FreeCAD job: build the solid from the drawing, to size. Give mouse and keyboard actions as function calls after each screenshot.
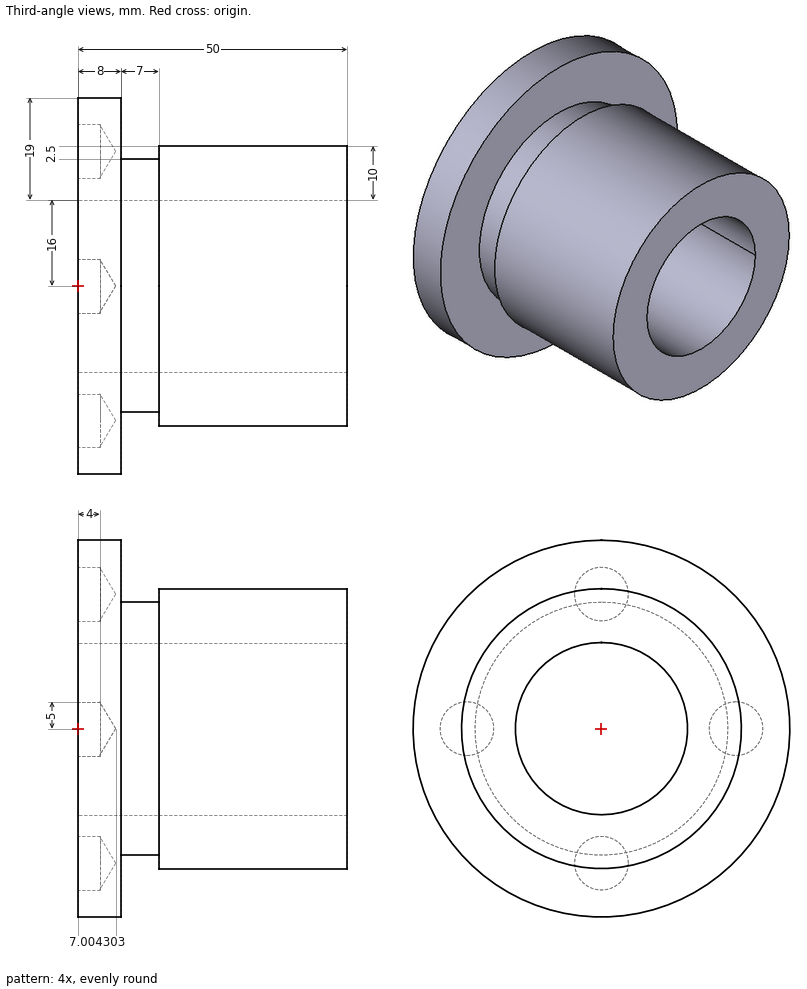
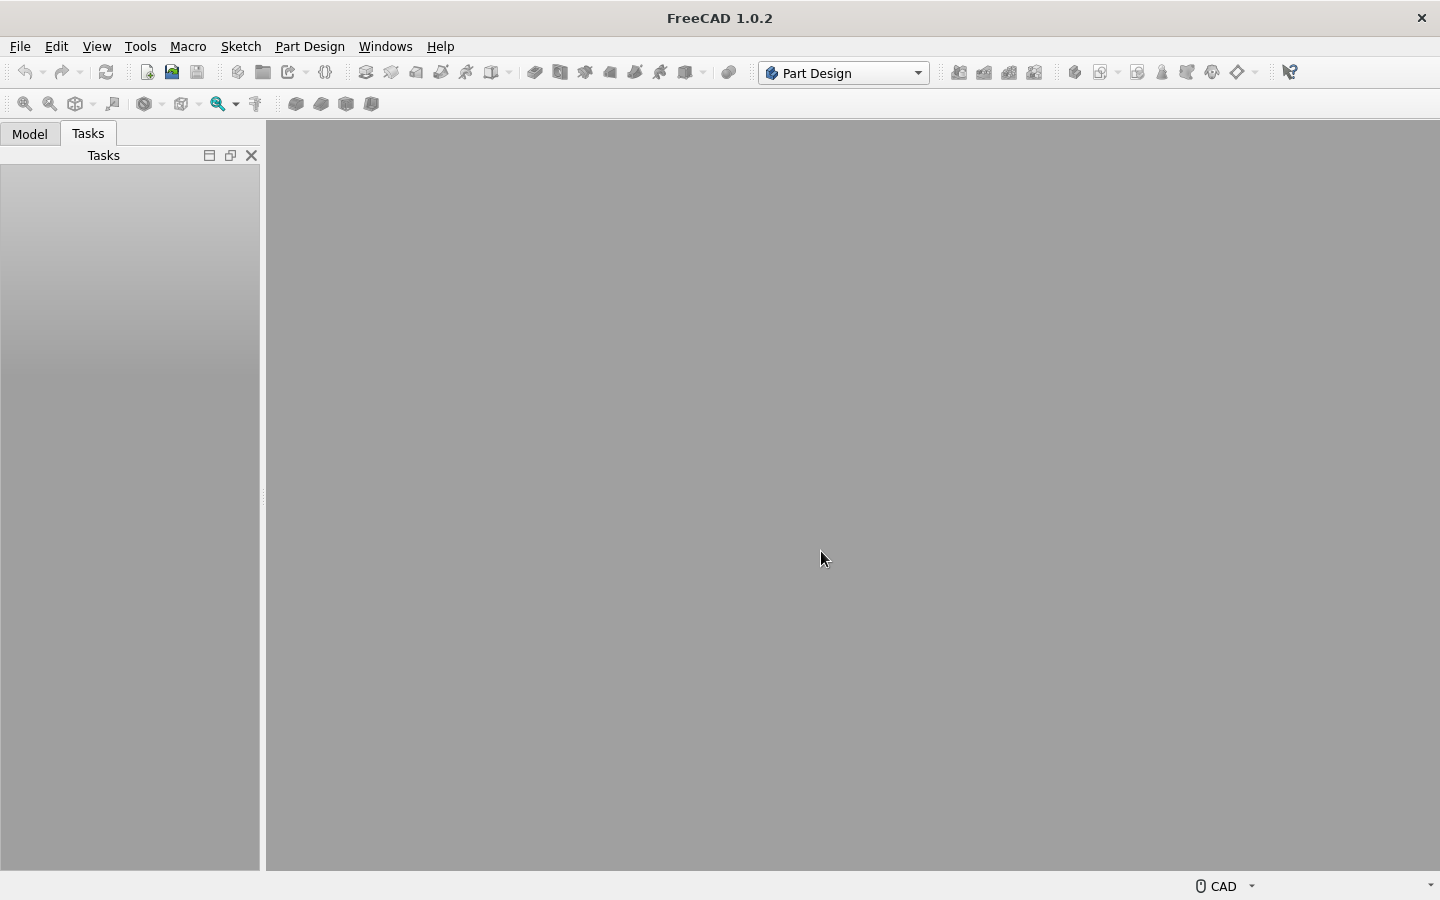
key(ctrl+n)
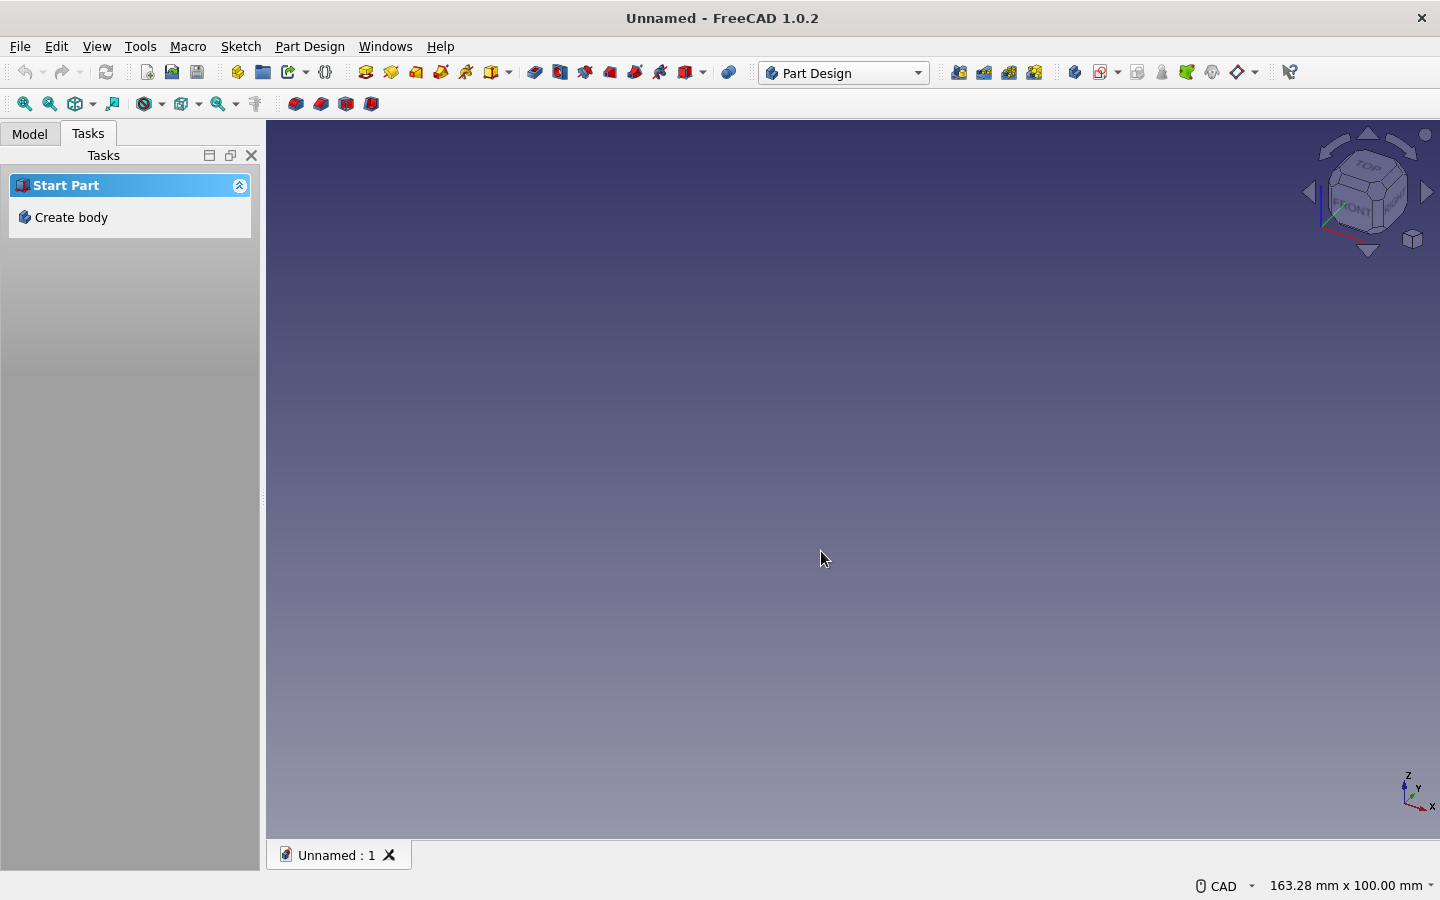
click(1100, 72)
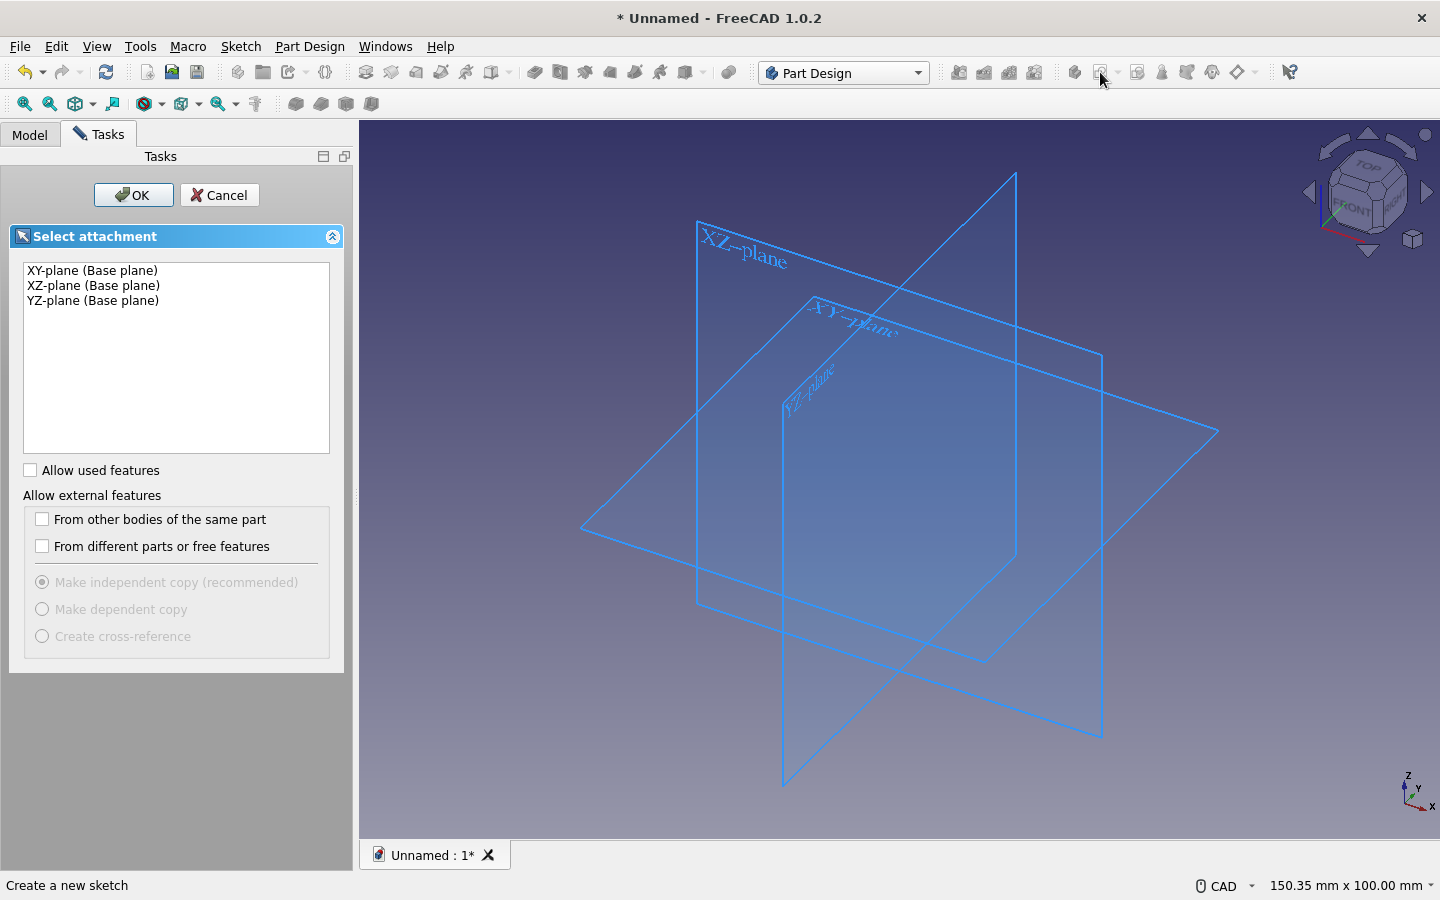
click(84, 270)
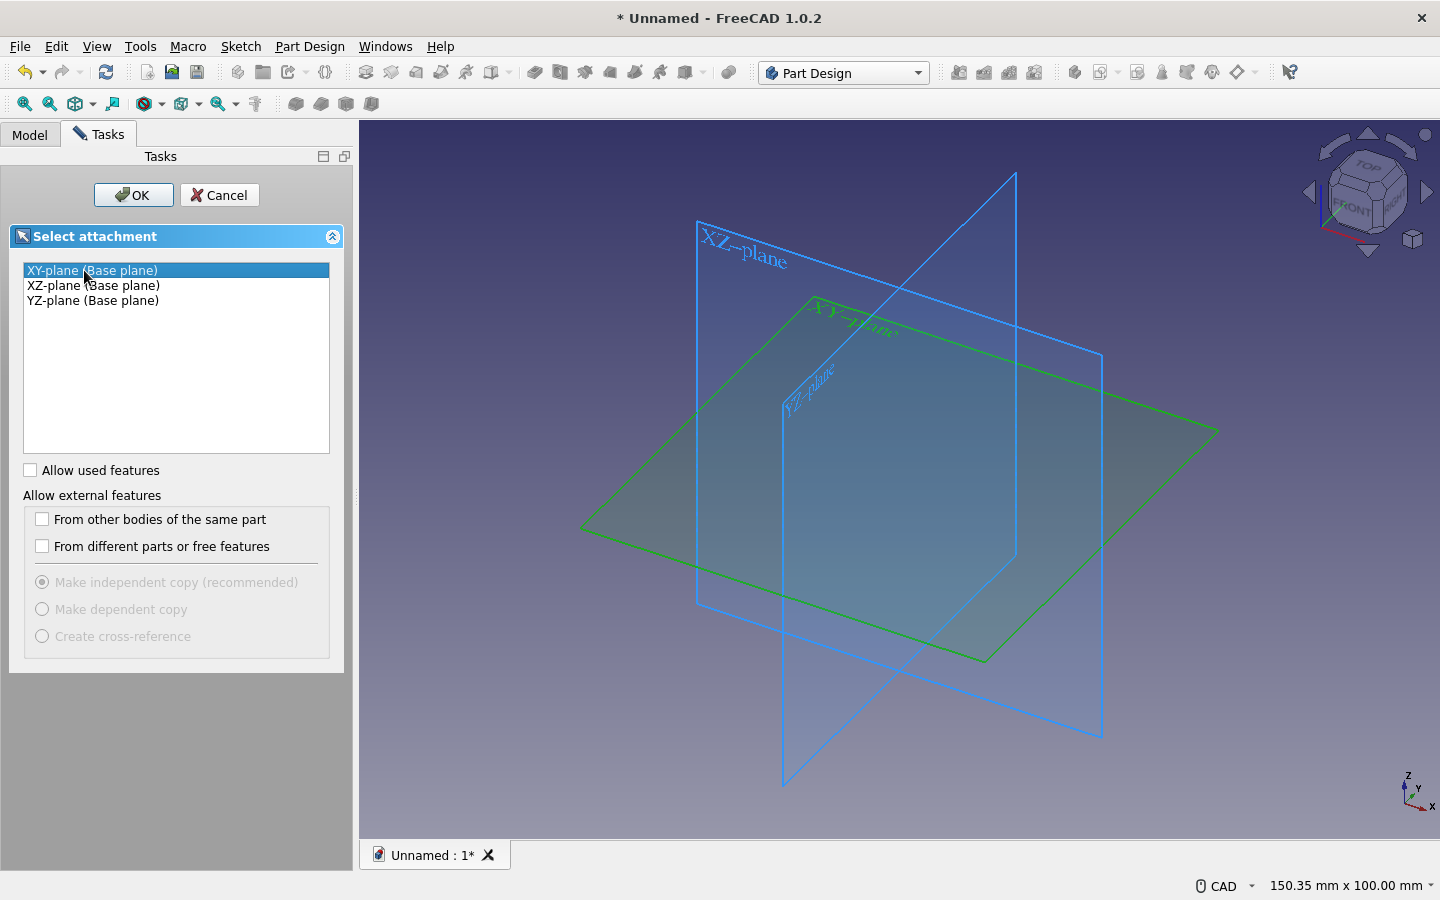
click(134, 195)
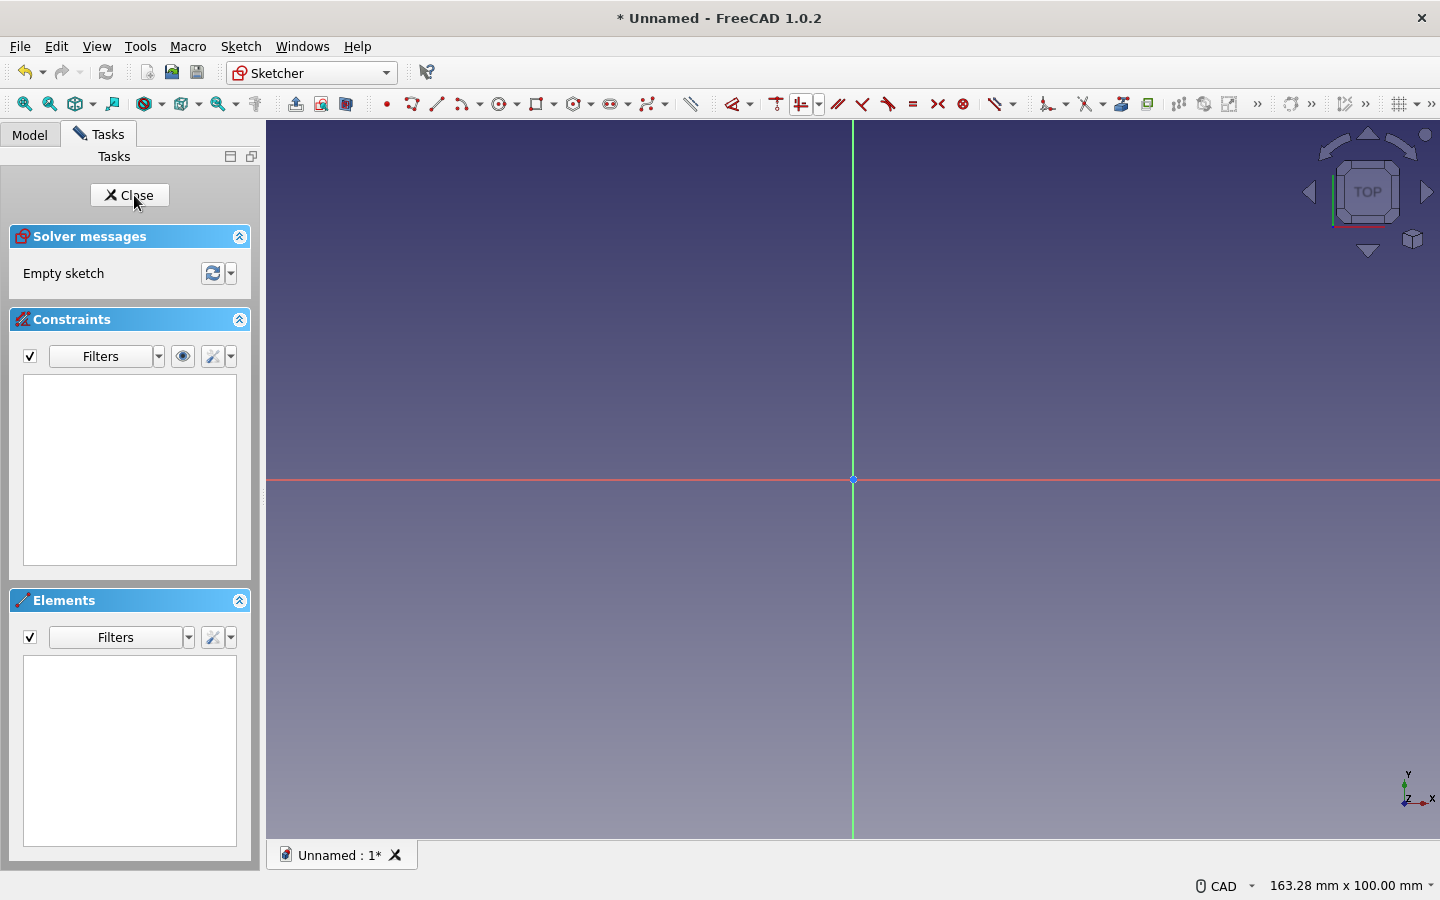
scroll(1275, 201, up, 3)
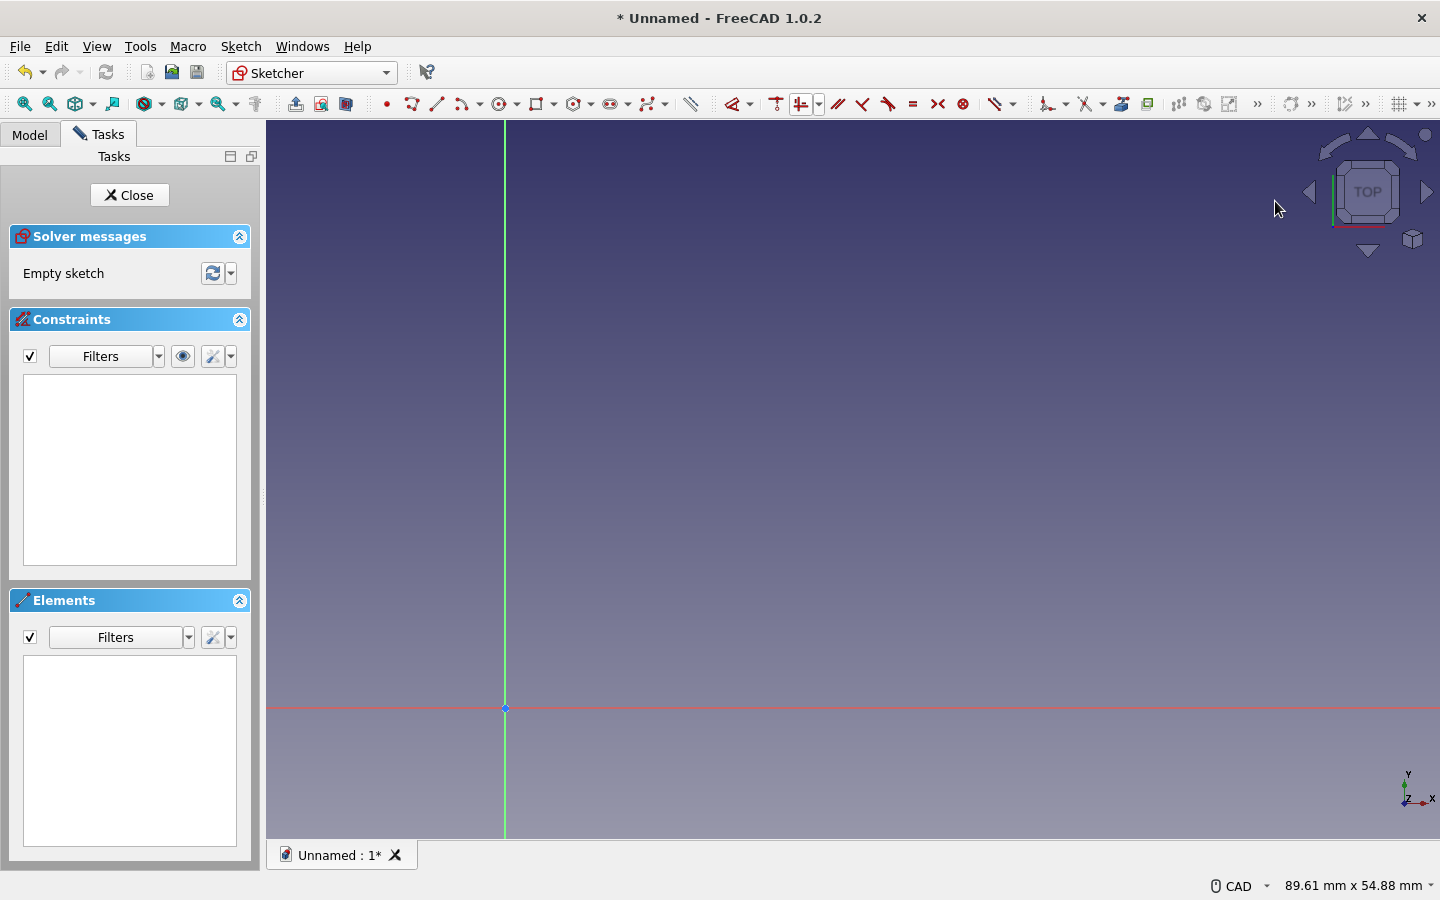
click(412, 104)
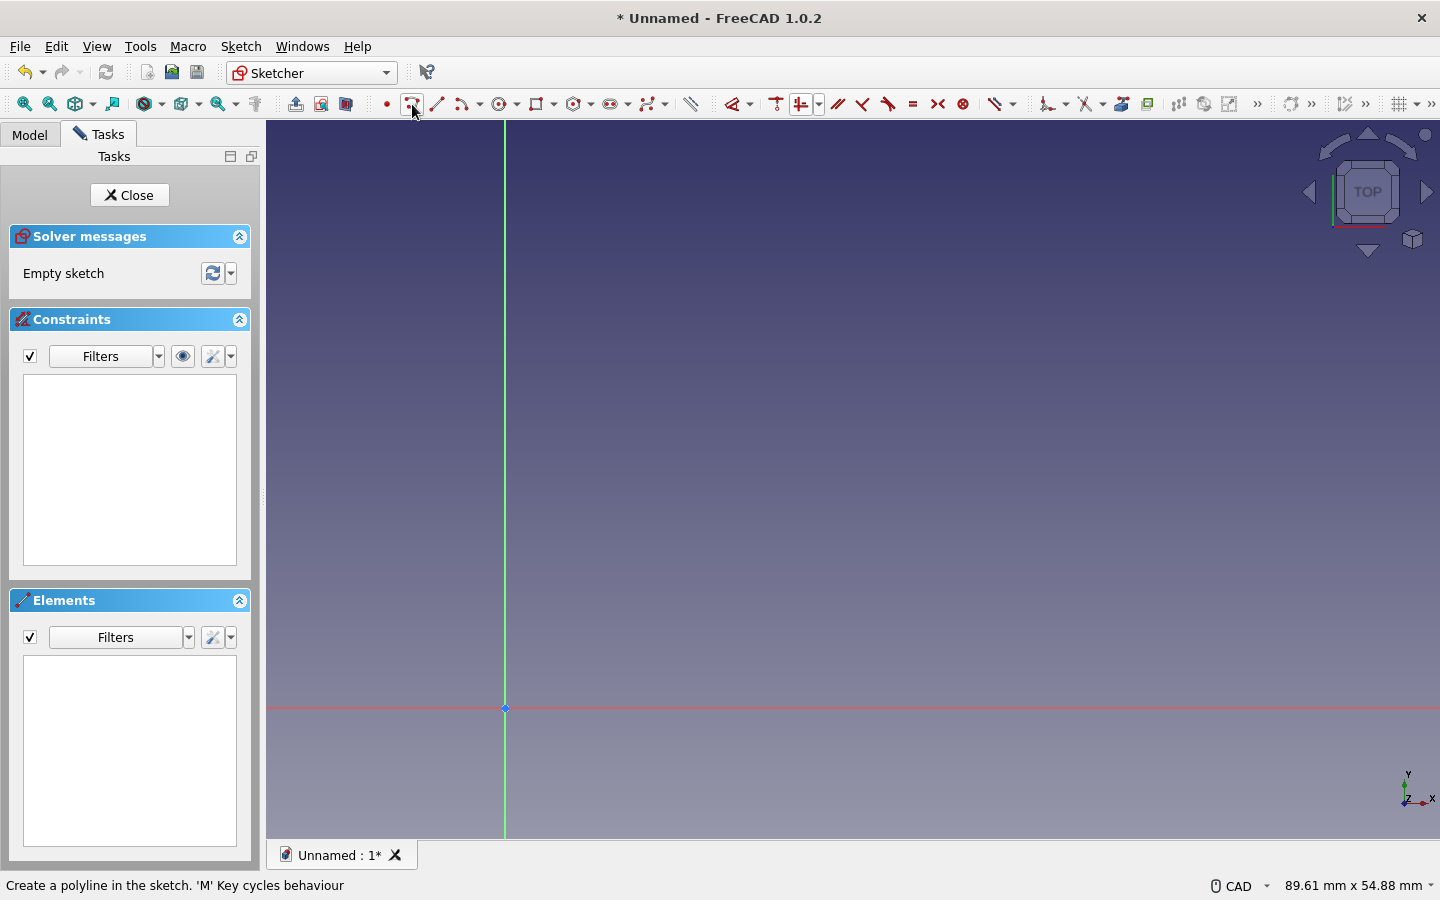
click(505, 499)
click(1160, 499)
click(1160, 368)
click(702, 368)
click(702, 400)
click(610, 400)
click(610, 250)
click(514, 250)
click(505, 500)
key(Escape)
key(Escape)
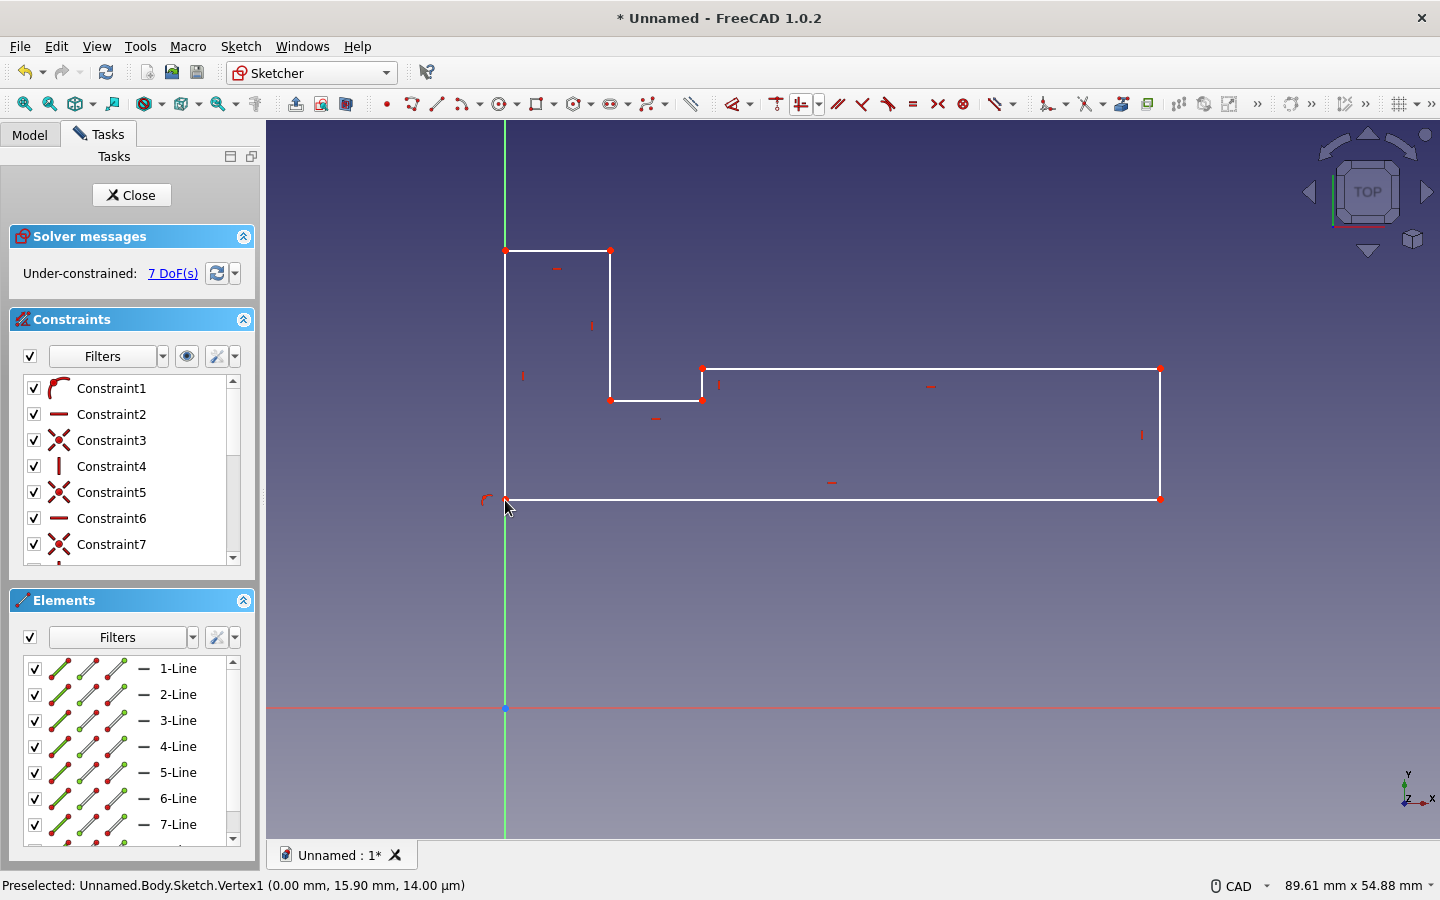
key(d)